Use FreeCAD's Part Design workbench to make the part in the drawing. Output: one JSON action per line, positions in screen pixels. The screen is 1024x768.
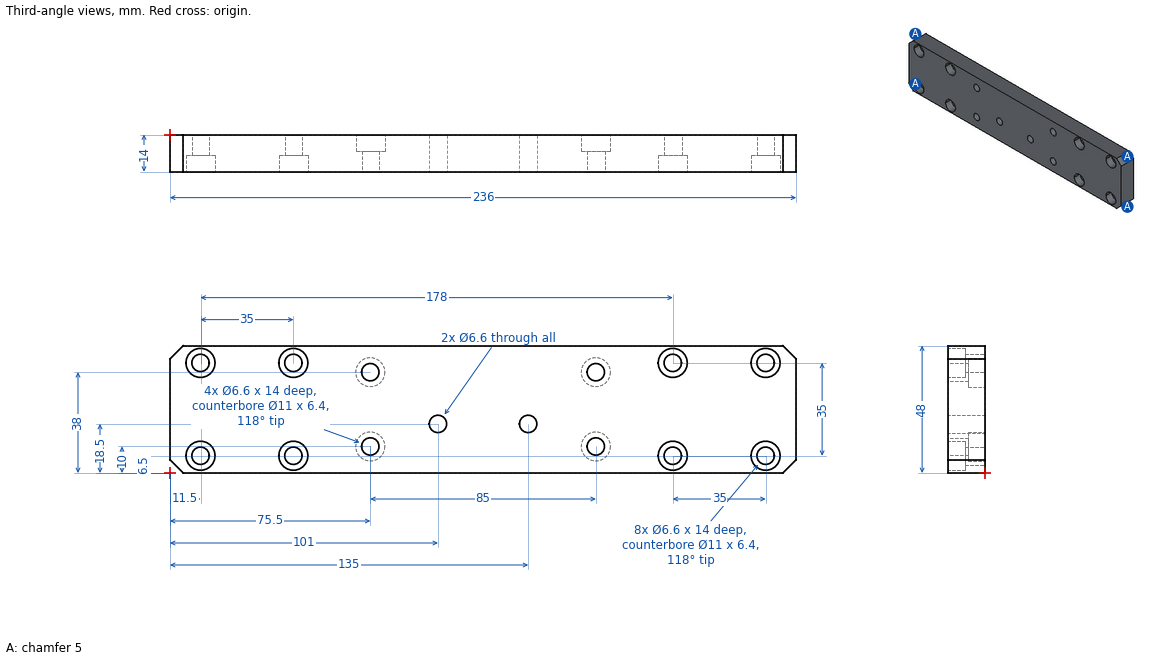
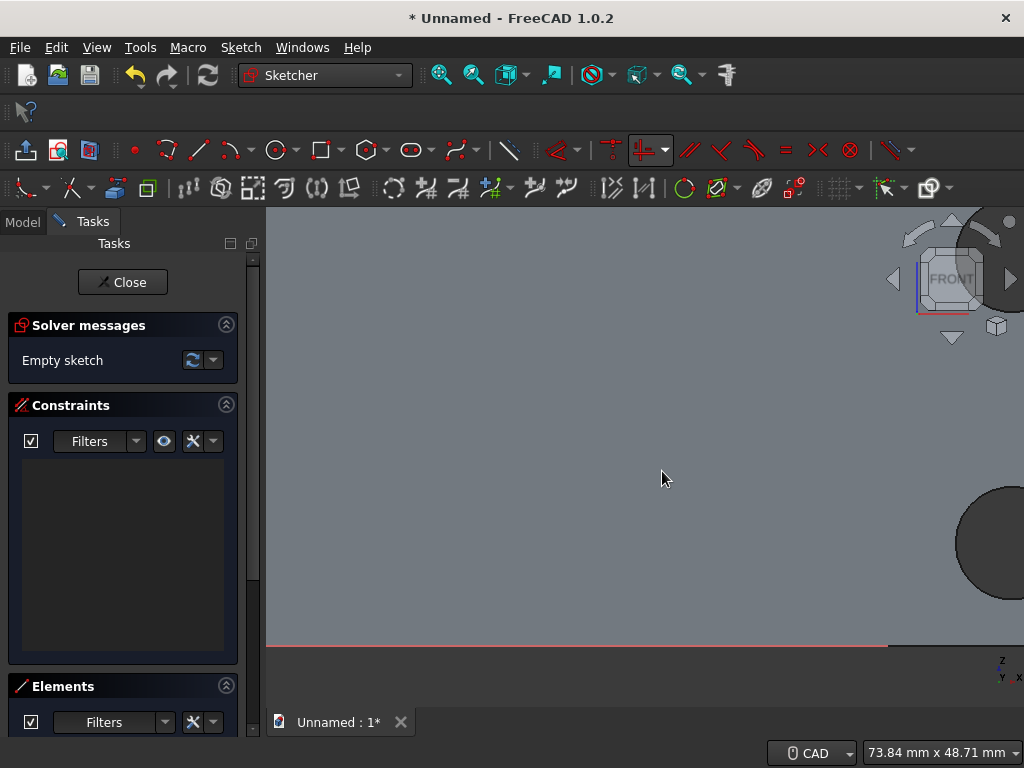
{"action": "left_click", "coordinate": [276, 150]}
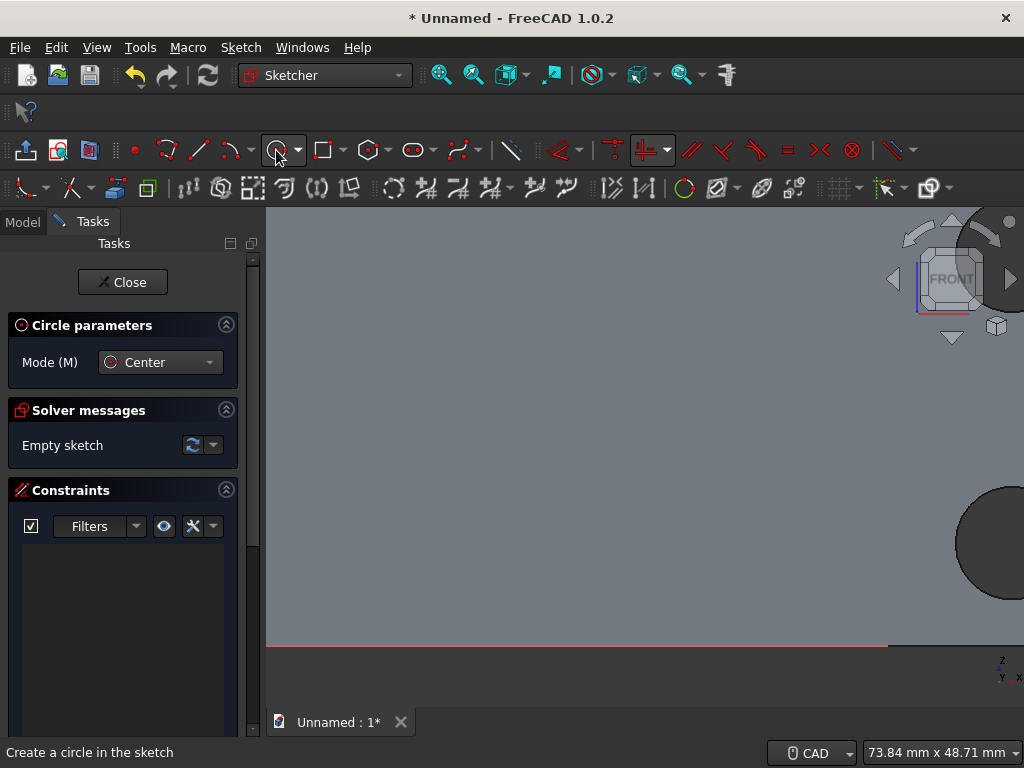
{"action": "left_click", "coordinate": [401, 456]}
{"action": "left_click", "coordinate": [425, 432]}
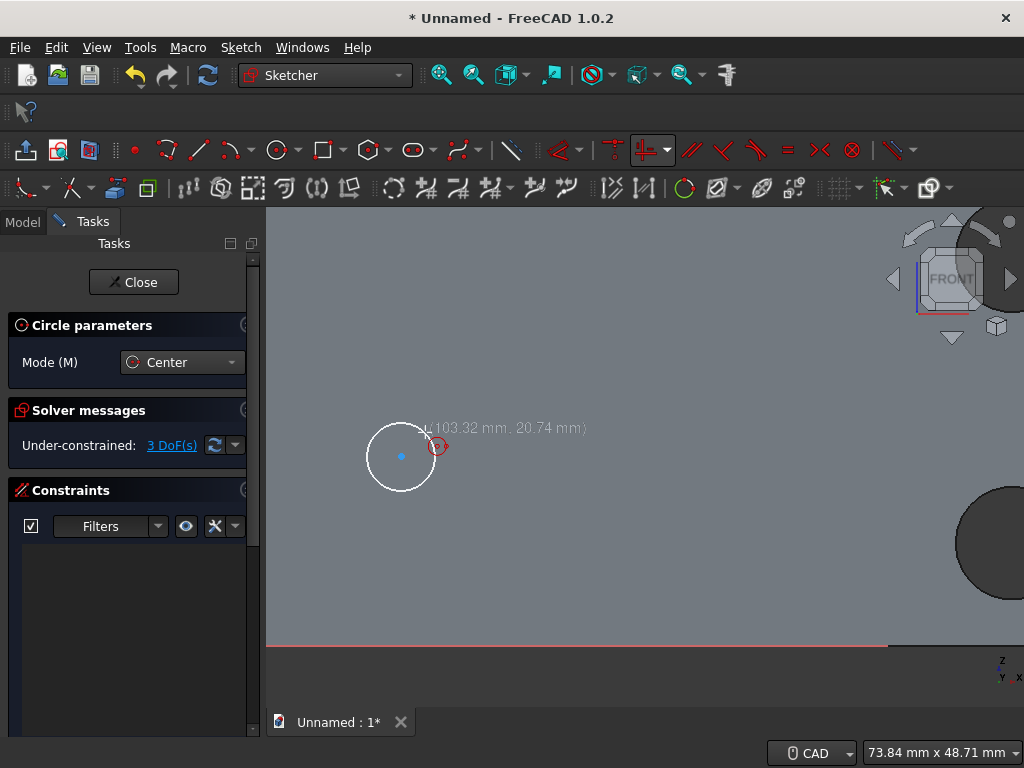
{"action": "left_click", "coordinate": [750, 456]}
{"action": "left_click", "coordinate": [774, 432]}
{"action": "key", "text": "Escape"}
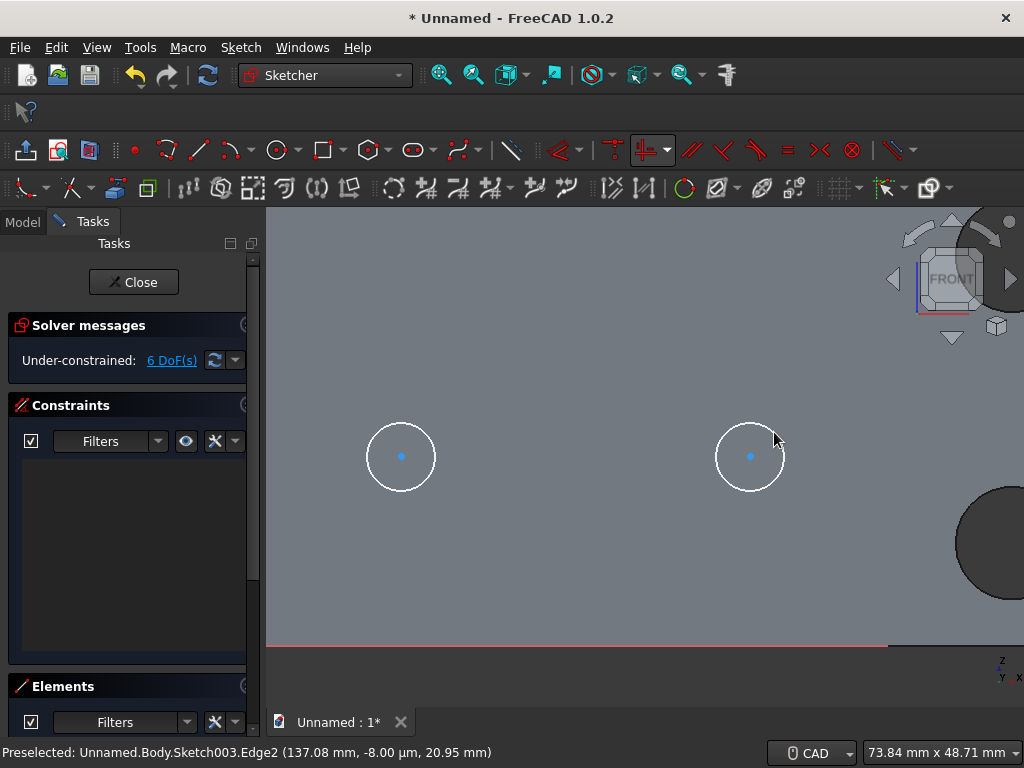
{"action": "left_click", "coordinate": [425, 433]}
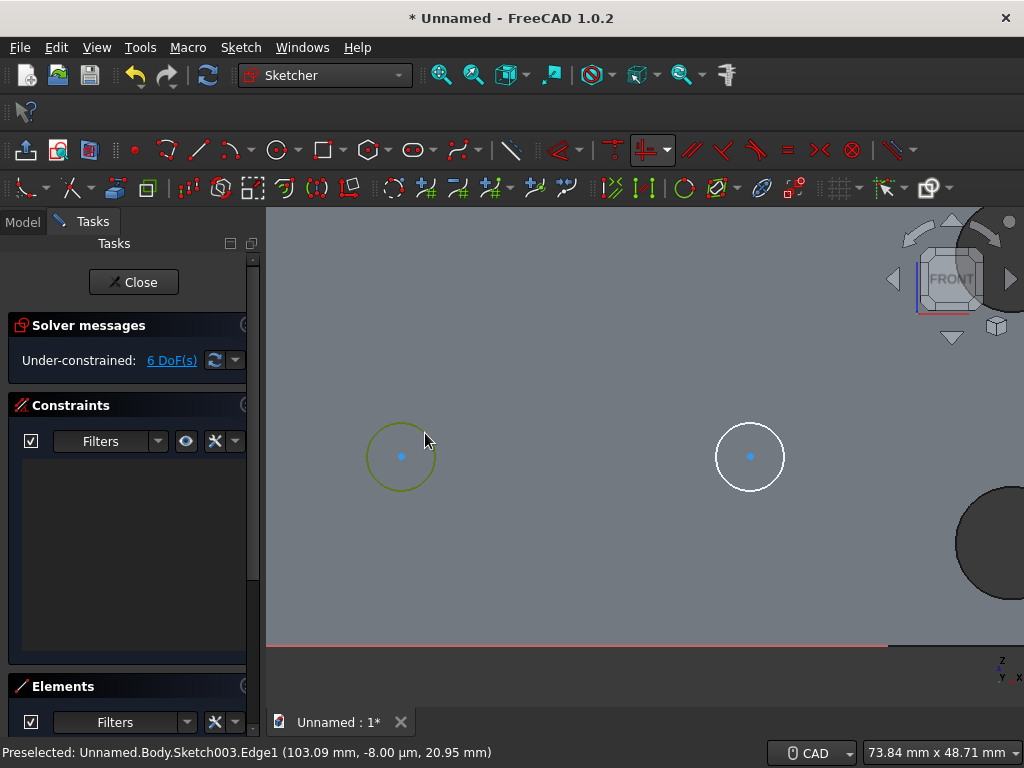
{"action": "left_click", "coordinate": [774, 433]}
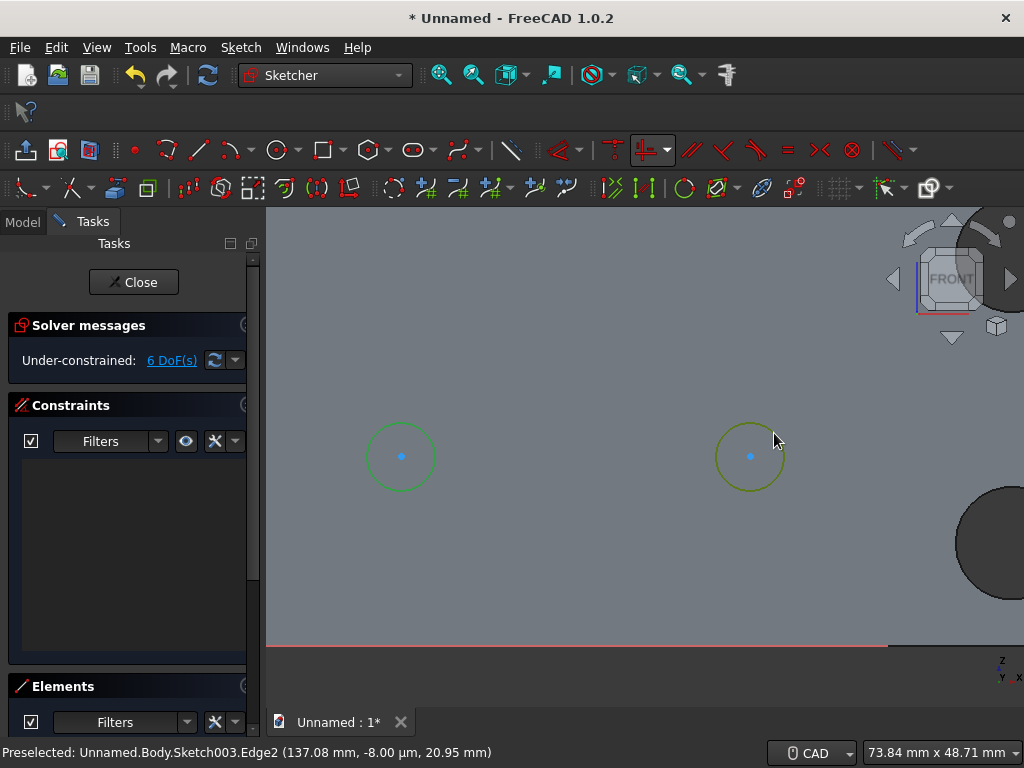
{"action": "left_click", "coordinate": [788, 150]}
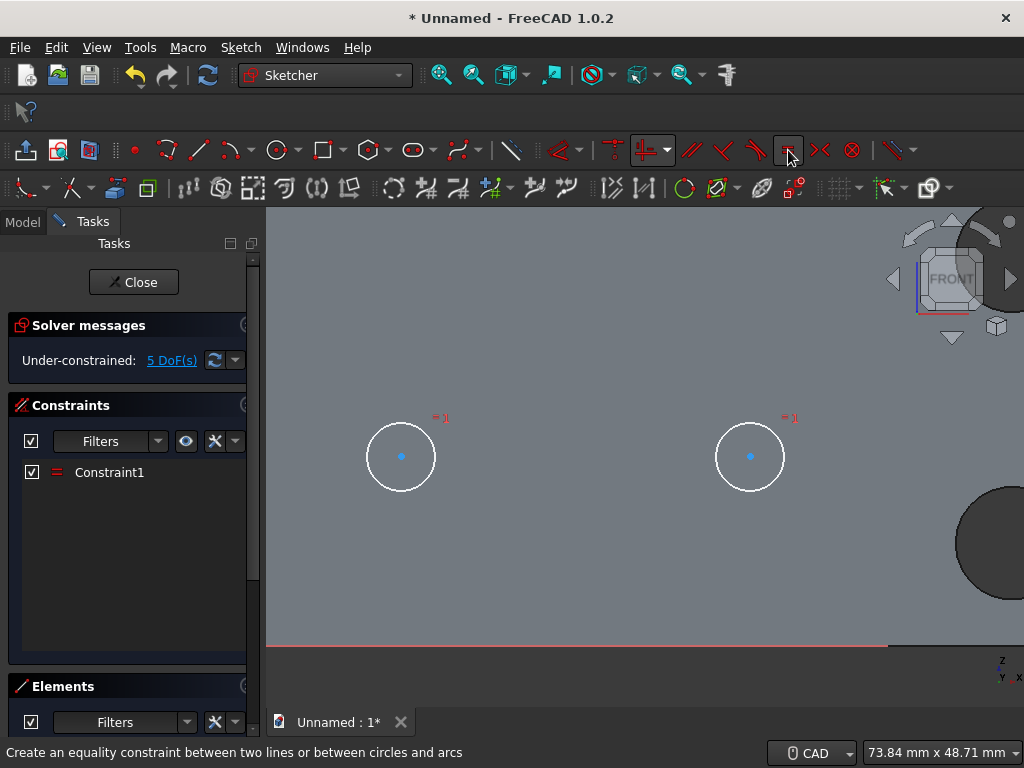
{"action": "left_click", "coordinate": [401, 457]}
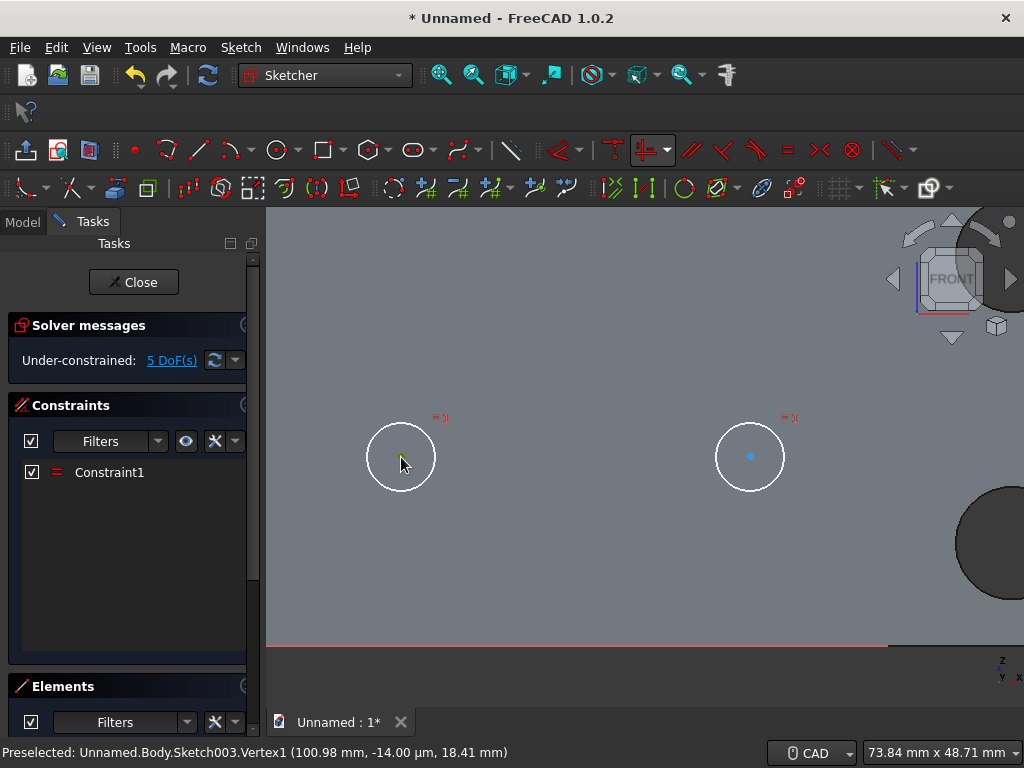
{"action": "left_click", "coordinate": [750, 457]}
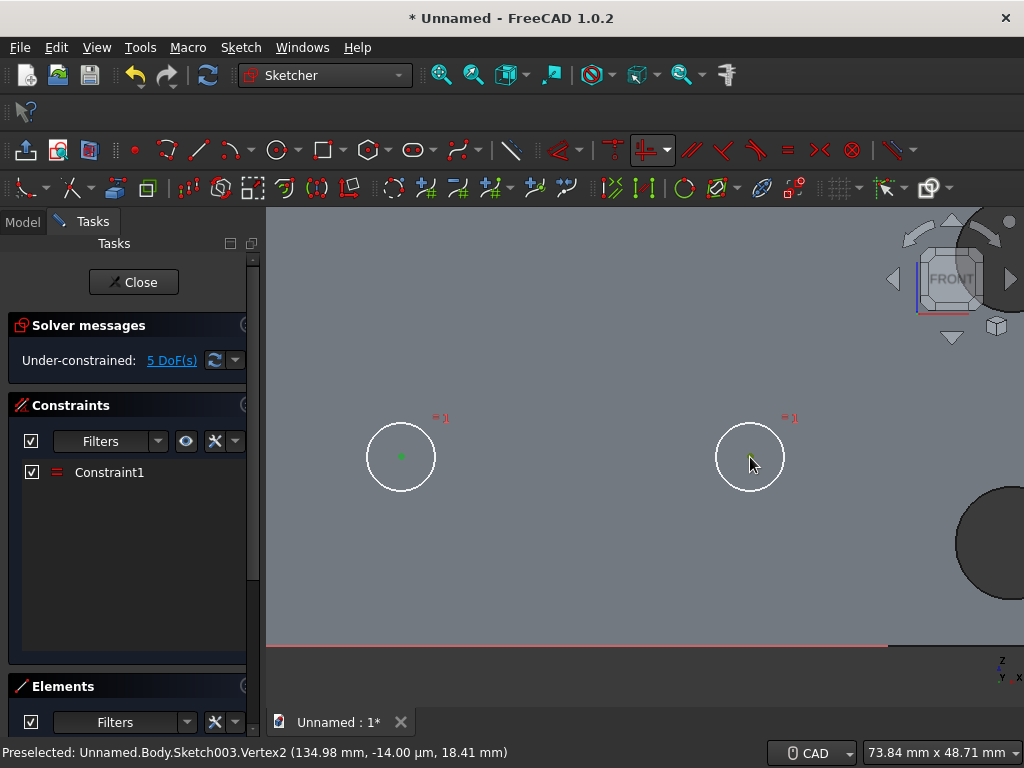
{"action": "left_click", "coordinate": [670, 150]}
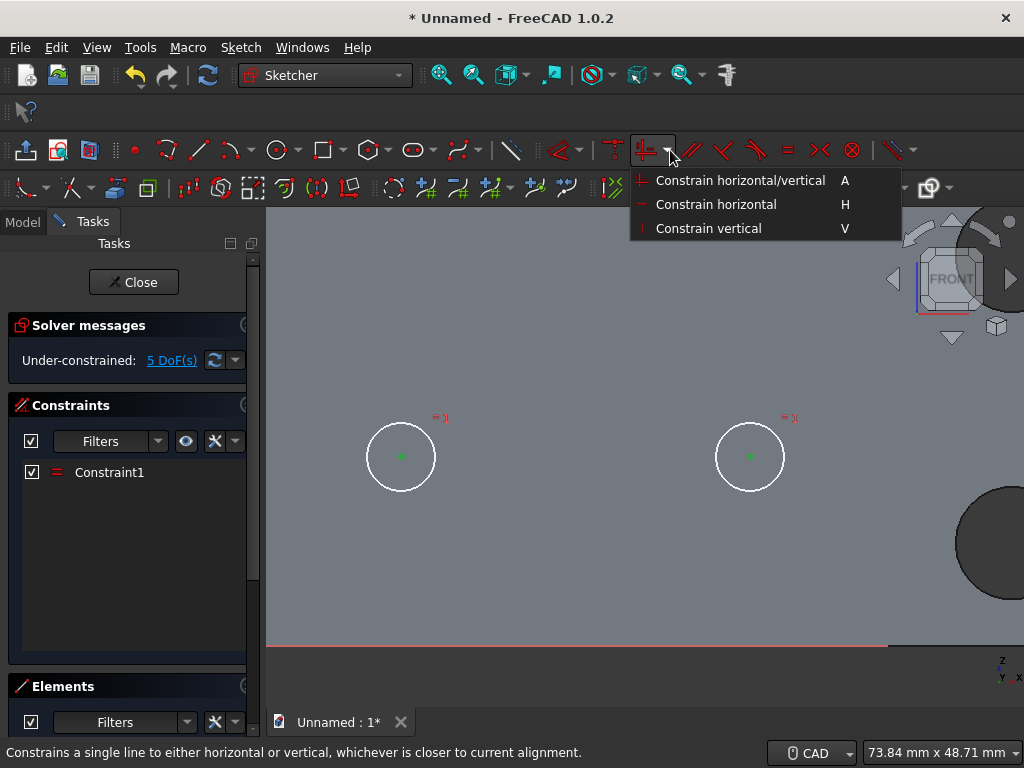
{"action": "left_click", "coordinate": [766, 204]}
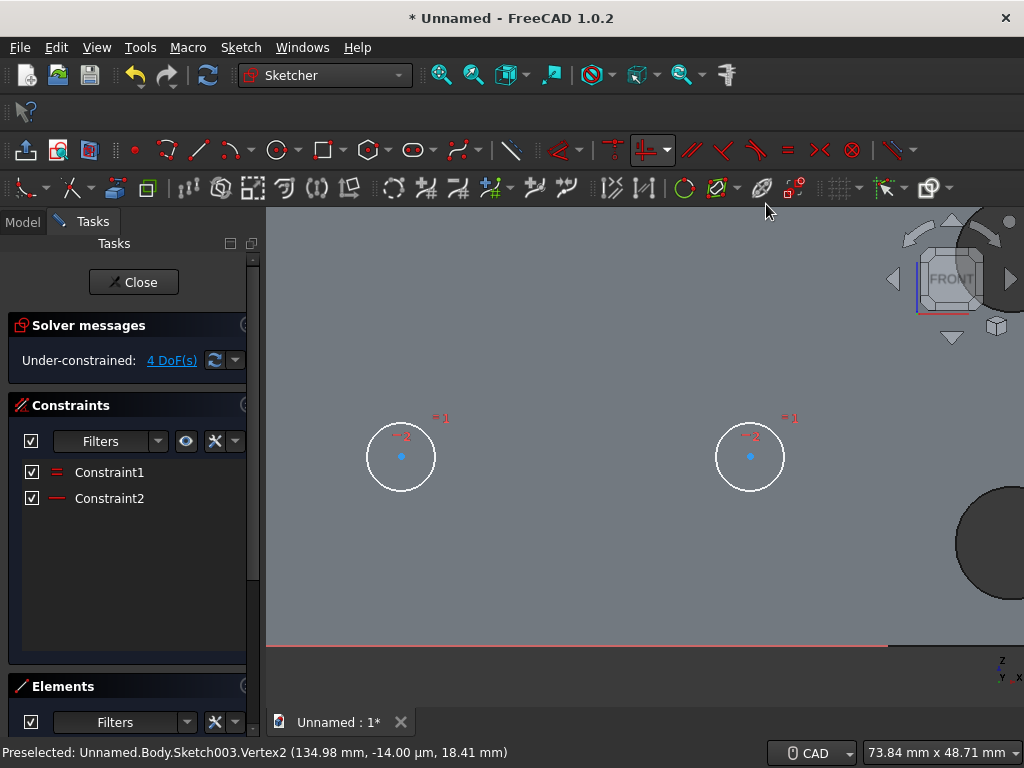
{"action": "left_click", "coordinate": [558, 150]}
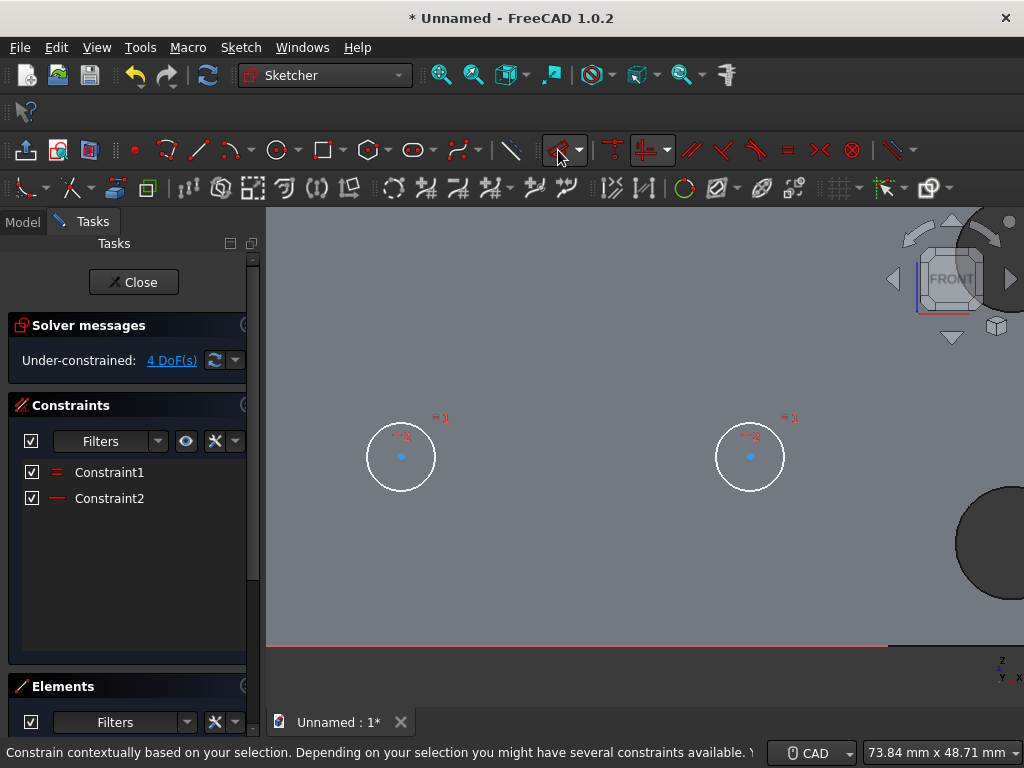
{"action": "left_click", "coordinate": [425, 433]}
{"action": "left_click", "coordinate": [448, 410]}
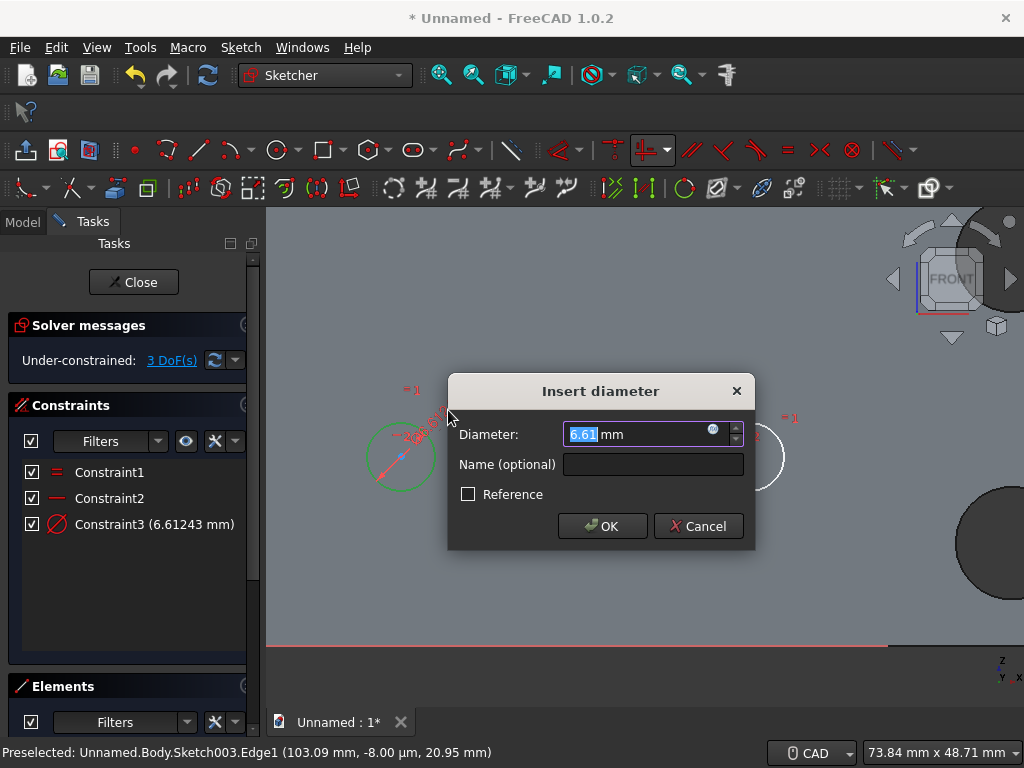
{"action": "type", "text": "6.6"}
{"action": "key", "text": "Return"}